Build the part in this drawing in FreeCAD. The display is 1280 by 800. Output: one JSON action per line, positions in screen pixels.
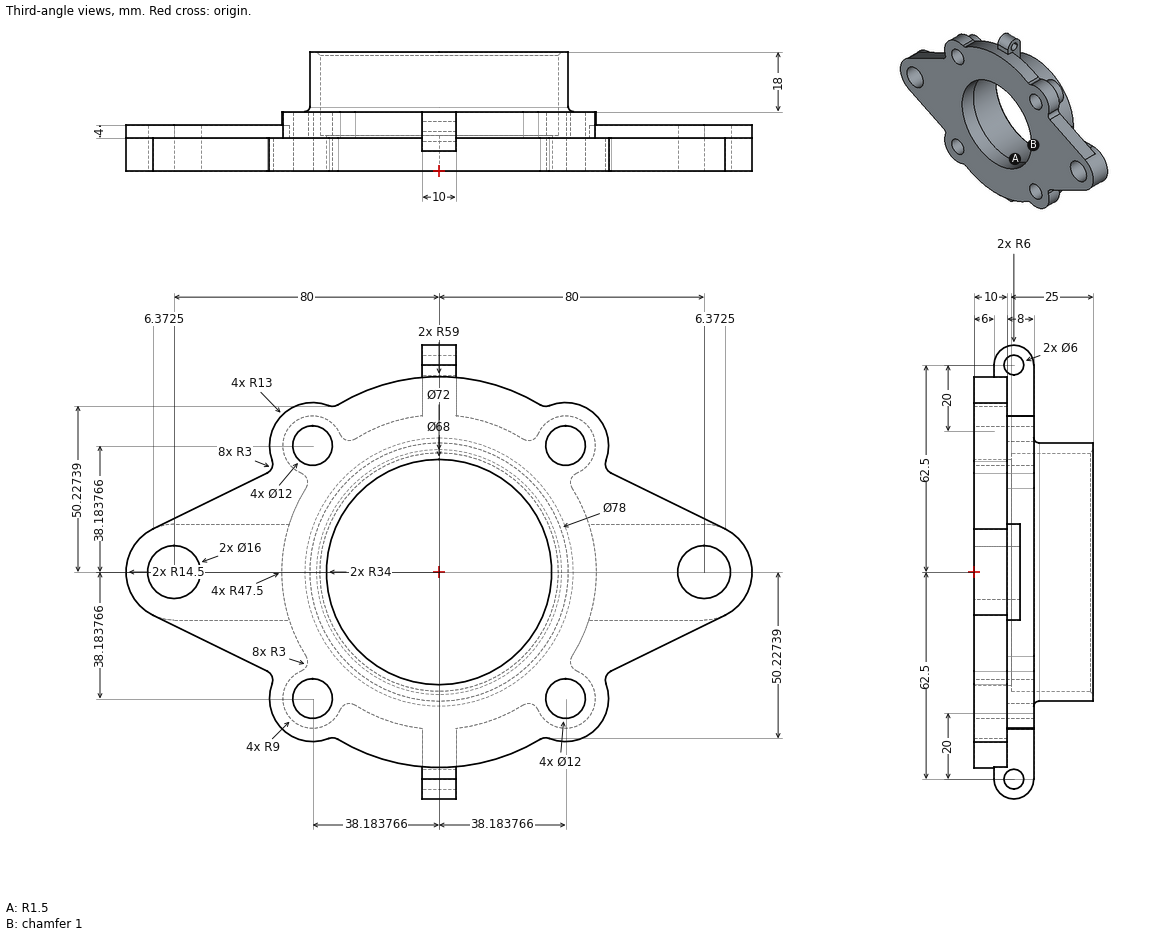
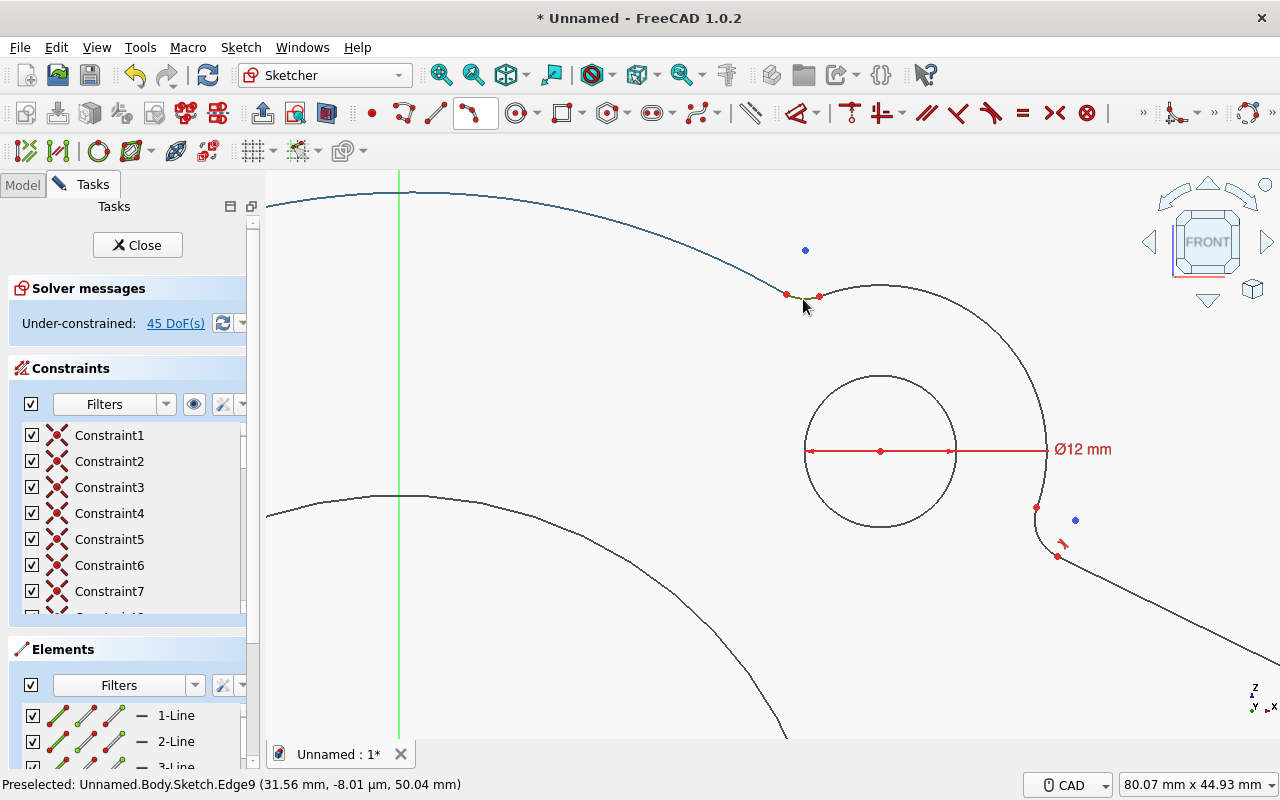
{"action": "left_click", "coordinate": [992, 114]}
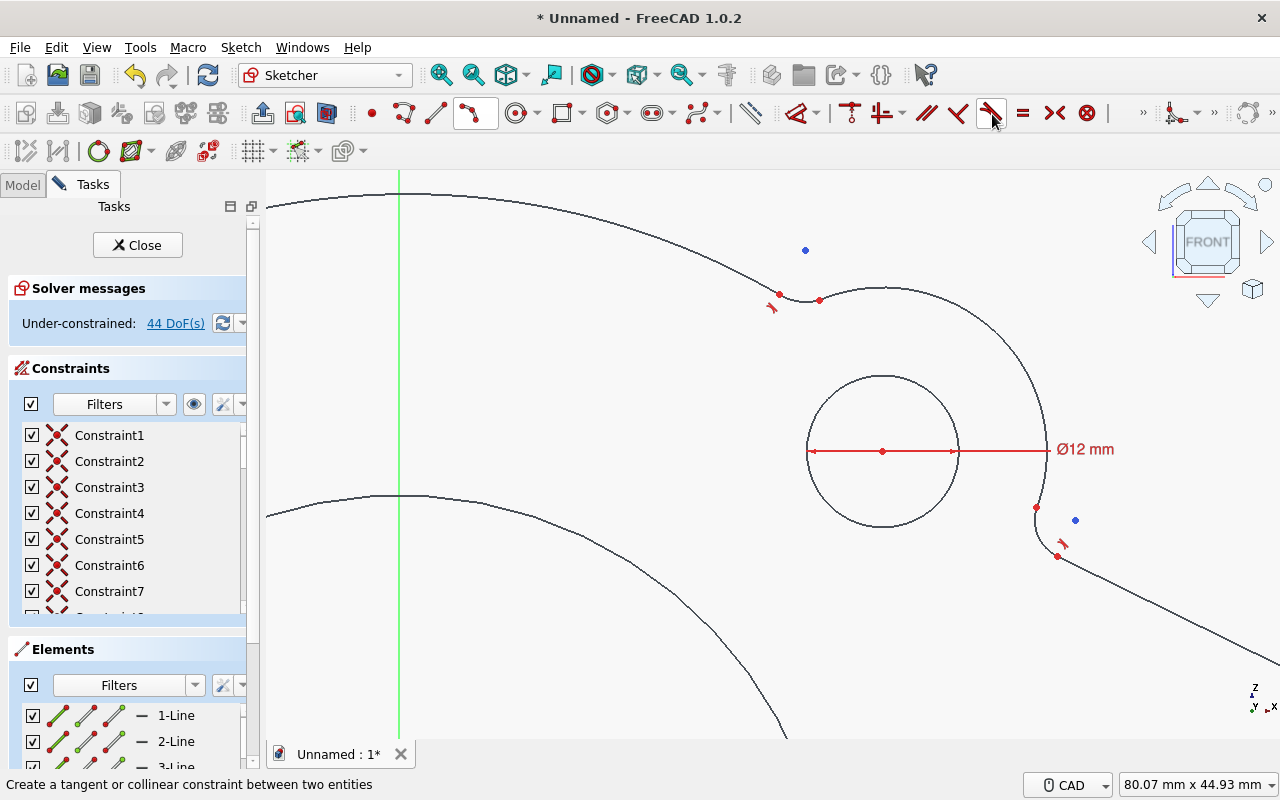
{"action": "left_click", "coordinate": [791, 300]}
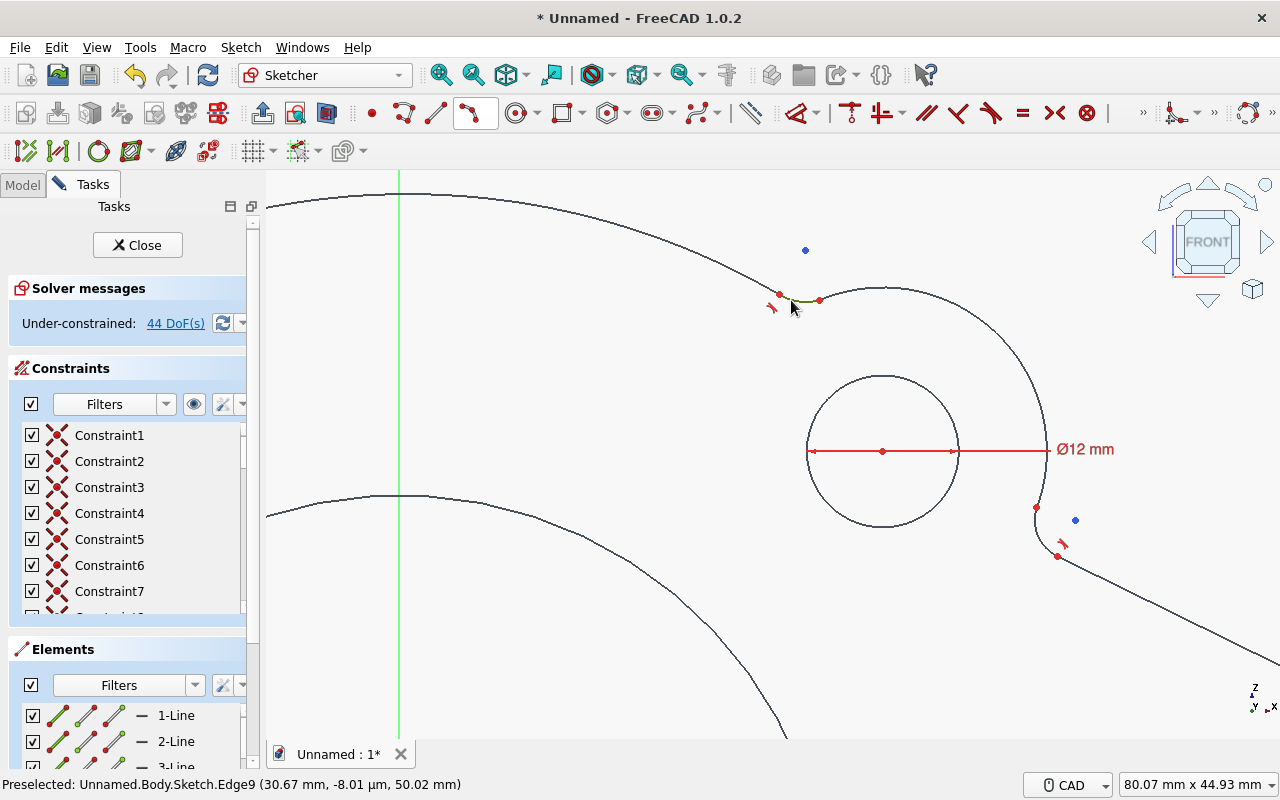
{"action": "scroll", "coordinate": [805, 298], "scroll_direction": "down", "scroll_amount": 7}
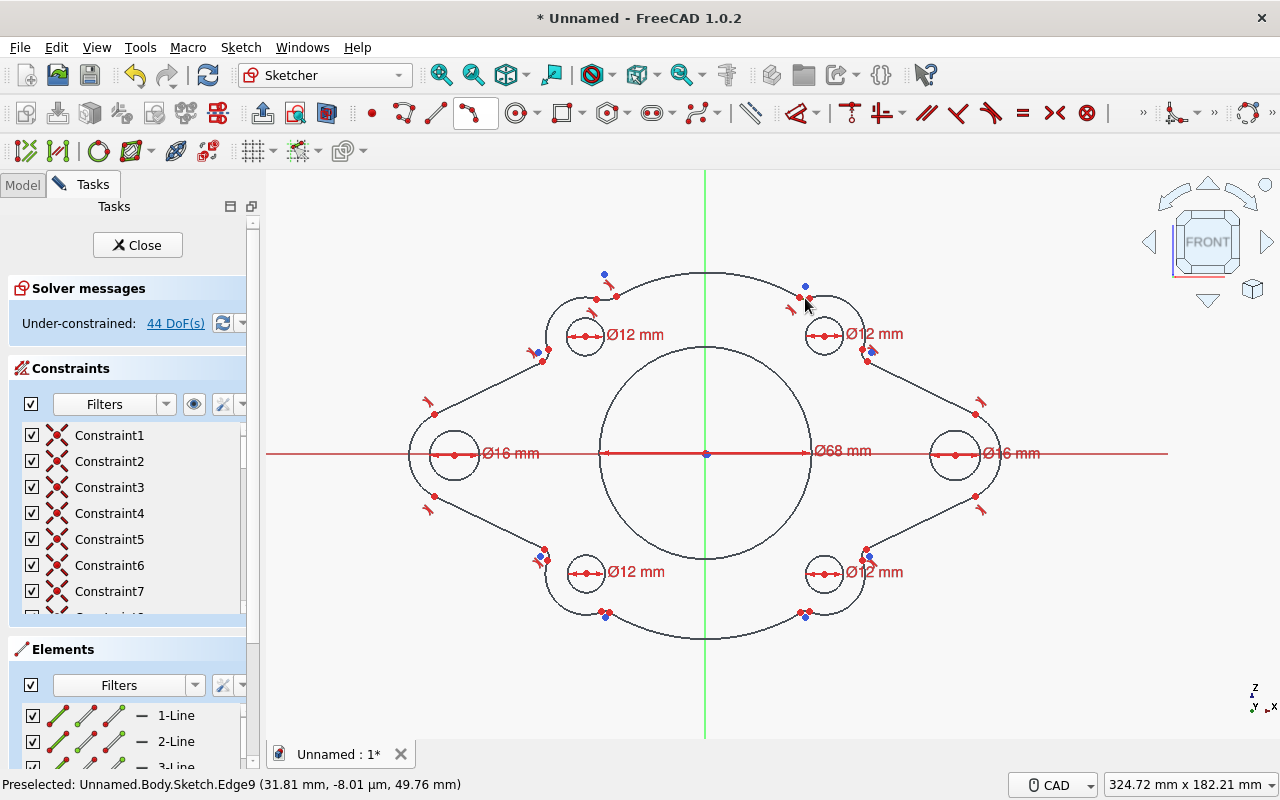
{"action": "left_click", "coordinate": [863, 322]}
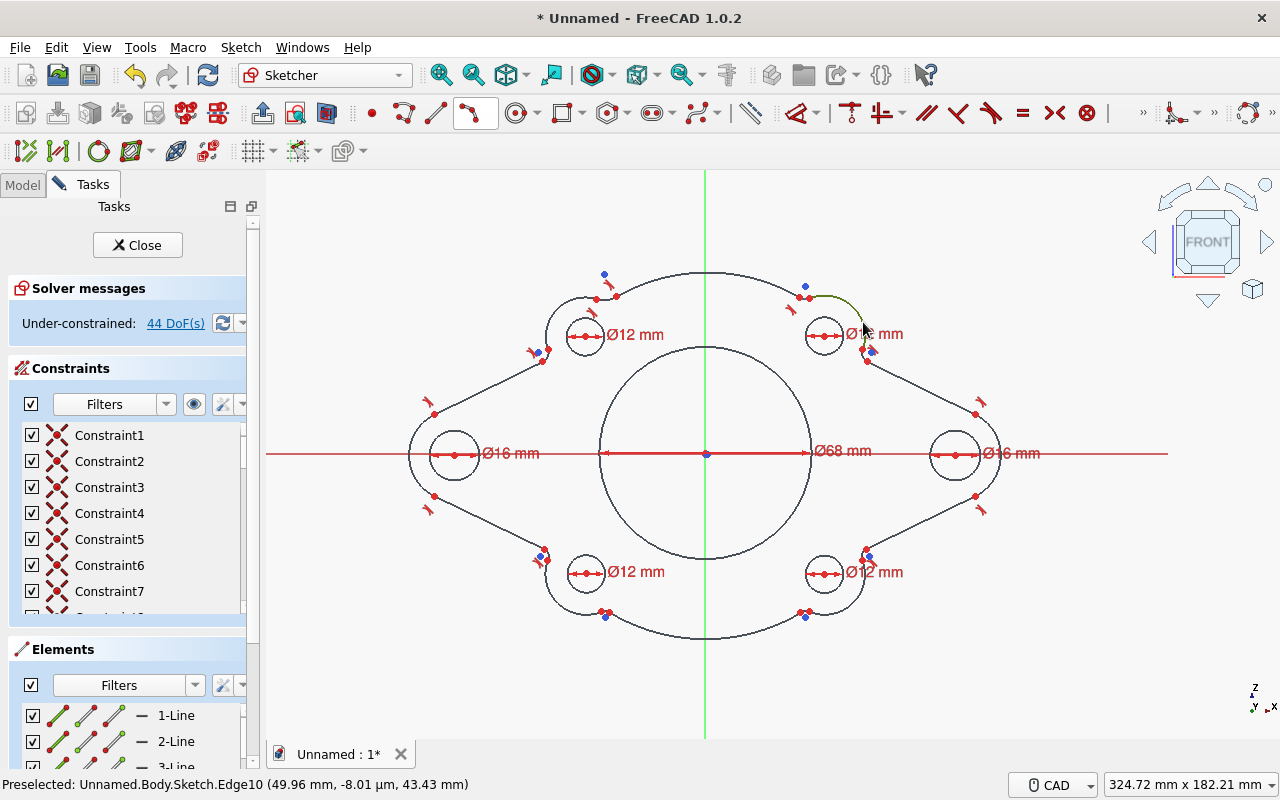
{"action": "left_click", "coordinate": [992, 114]}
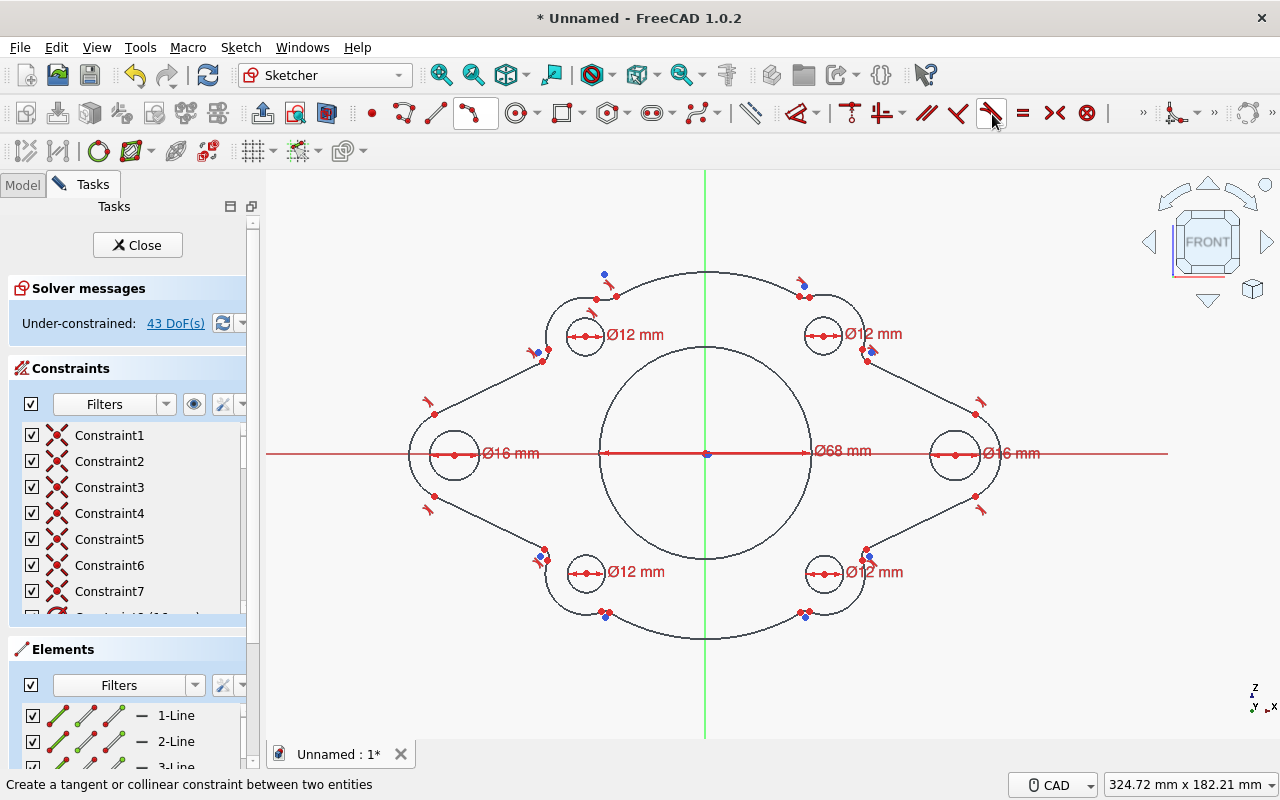
{"action": "left_click", "coordinate": [863, 322]}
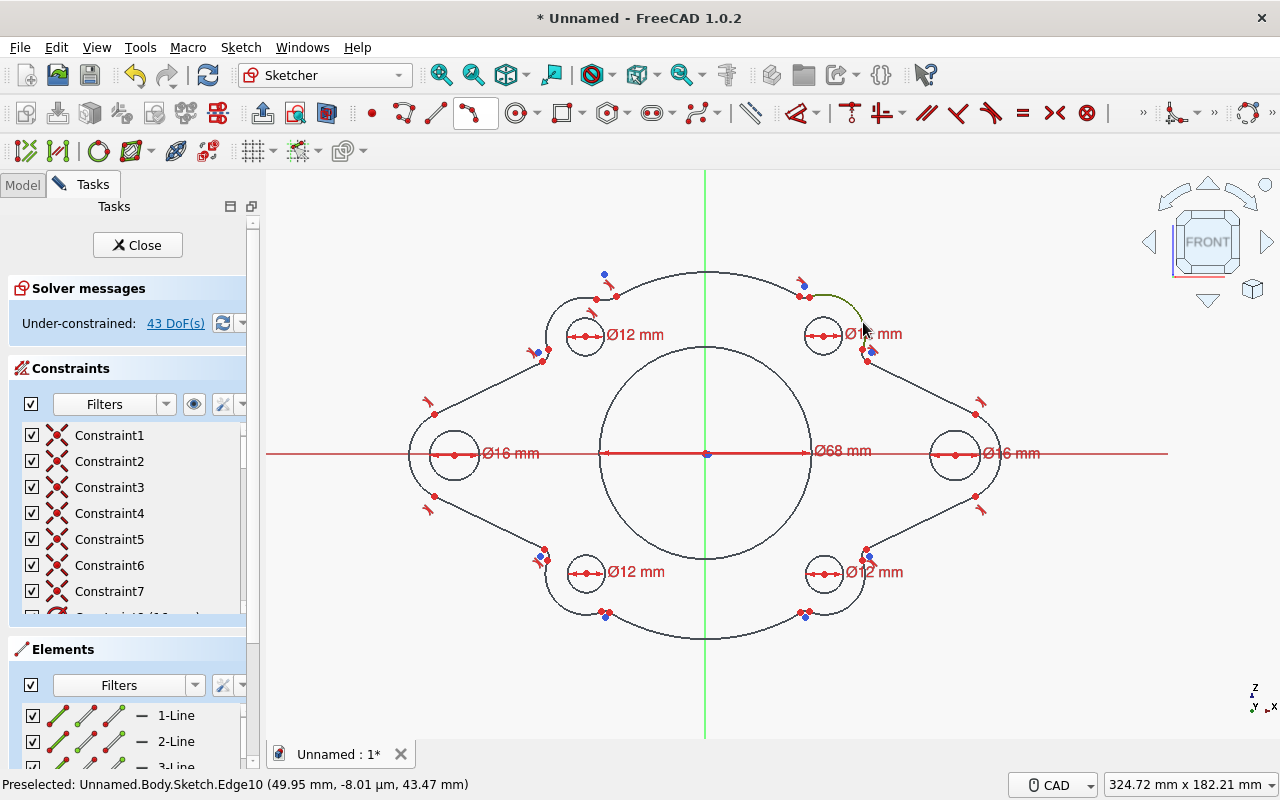
{"action": "scroll", "coordinate": [863, 357], "scroll_direction": "up", "scroll_amount": 4}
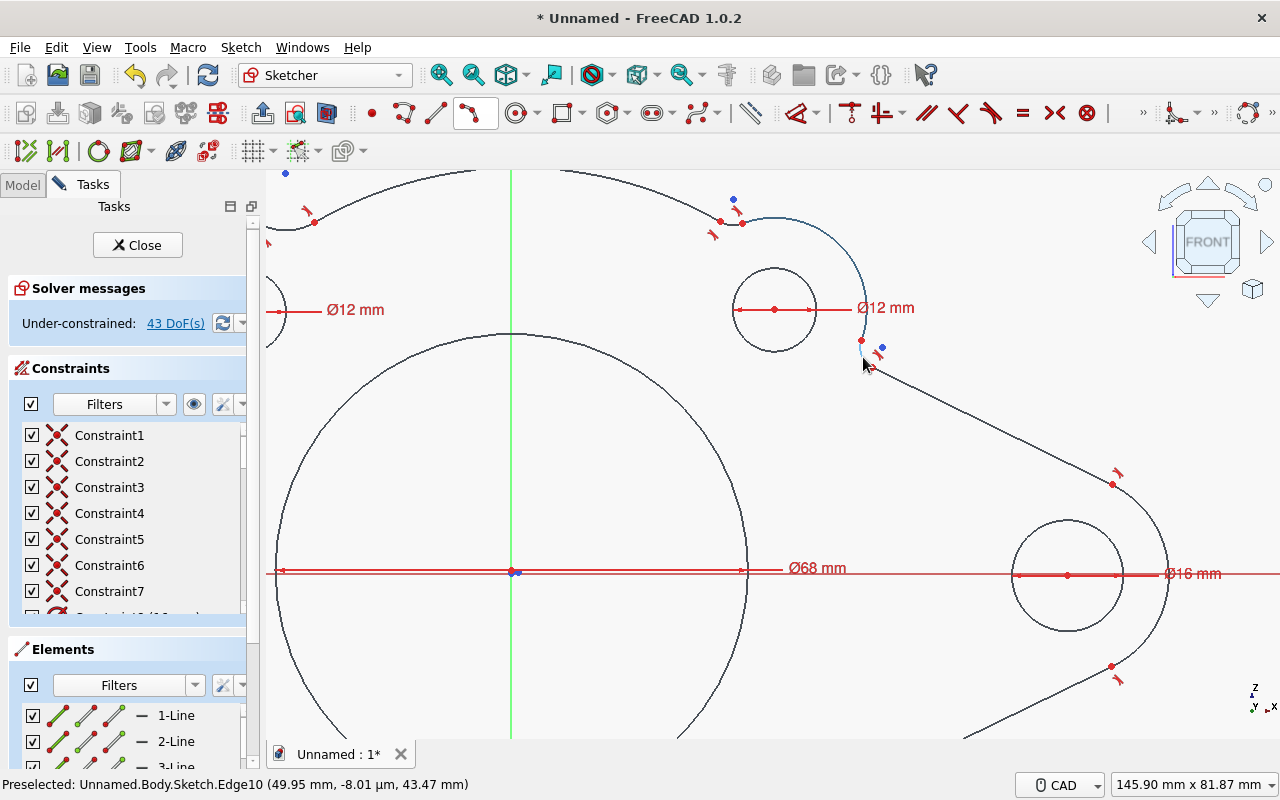
{"action": "left_click", "coordinate": [862, 356]}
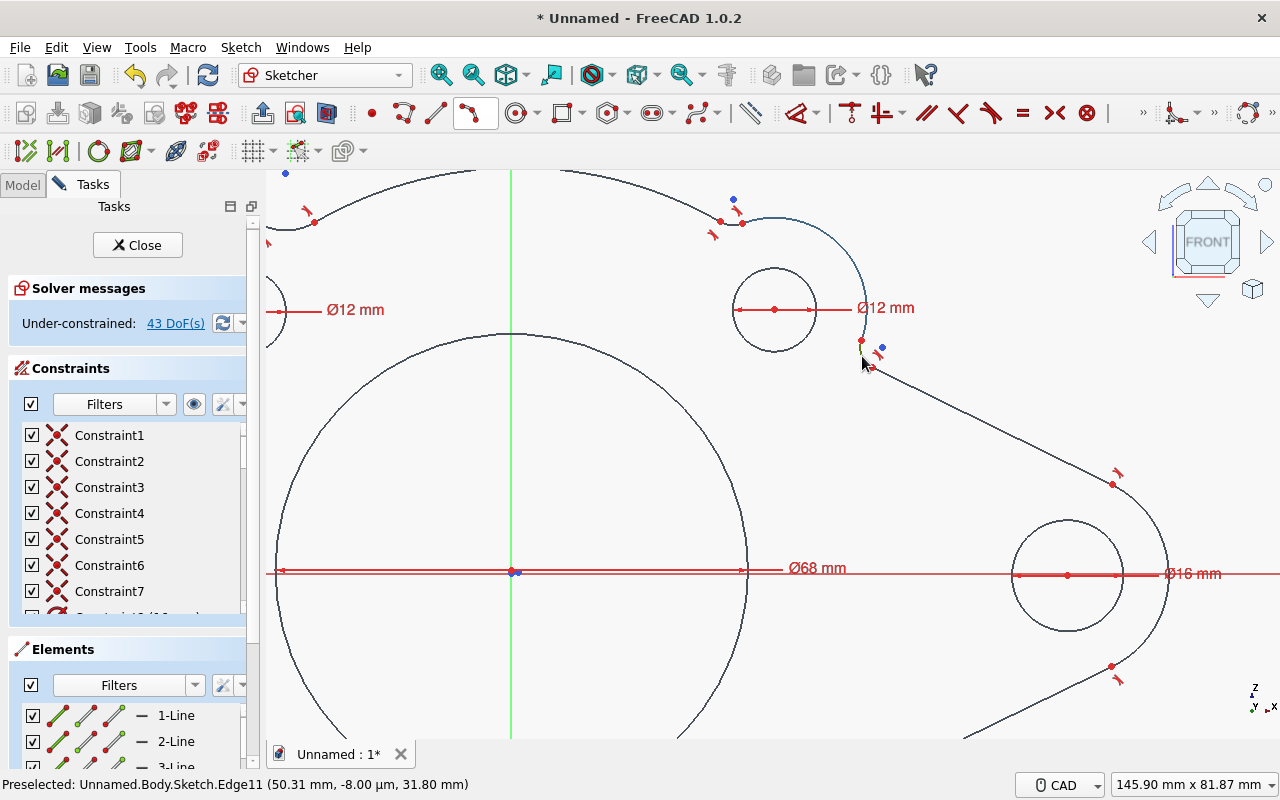
{"action": "left_click", "coordinate": [992, 114]}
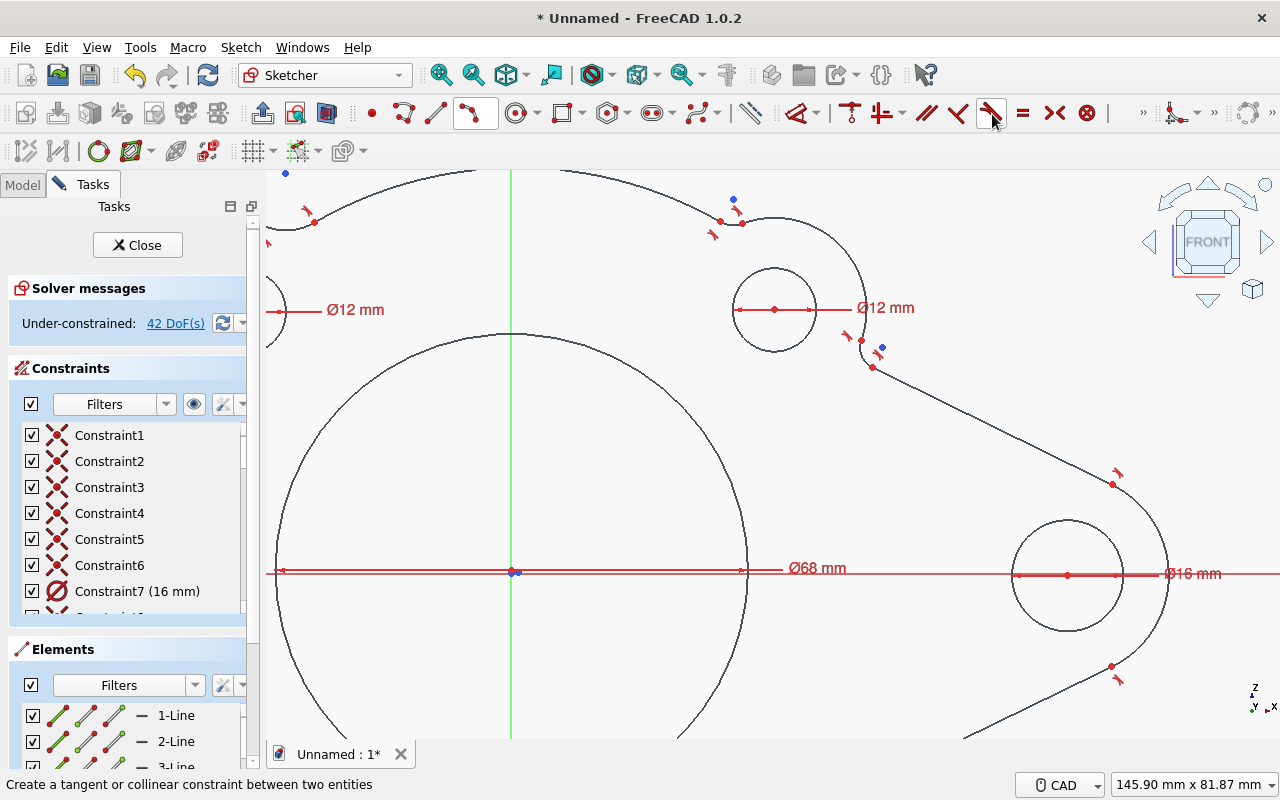
{"action": "scroll", "coordinate": [862, 357], "scroll_direction": "down", "scroll_amount": 4}